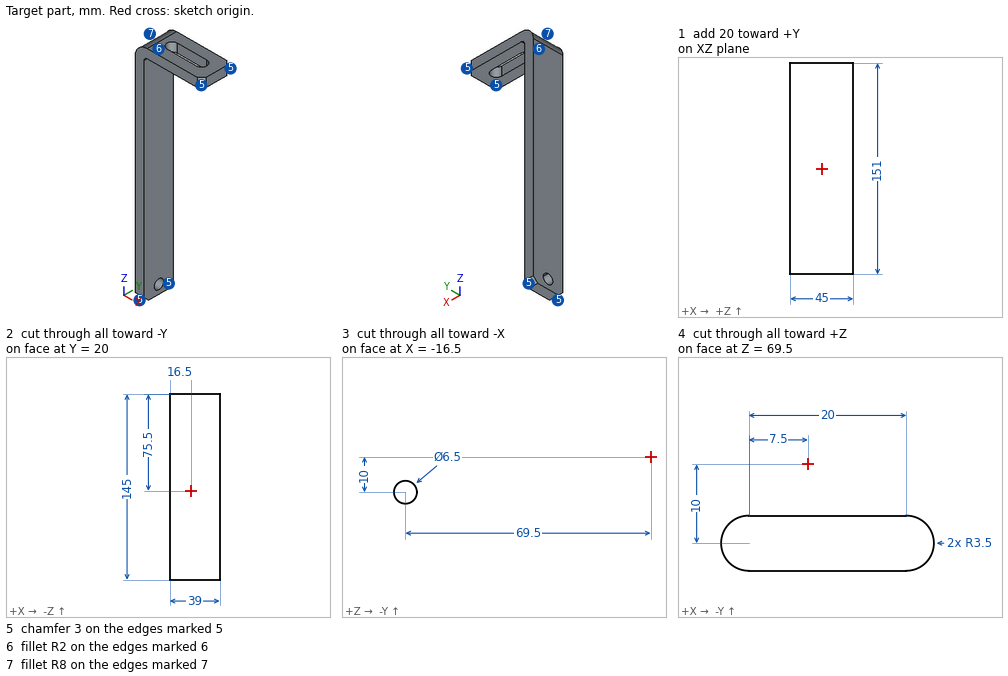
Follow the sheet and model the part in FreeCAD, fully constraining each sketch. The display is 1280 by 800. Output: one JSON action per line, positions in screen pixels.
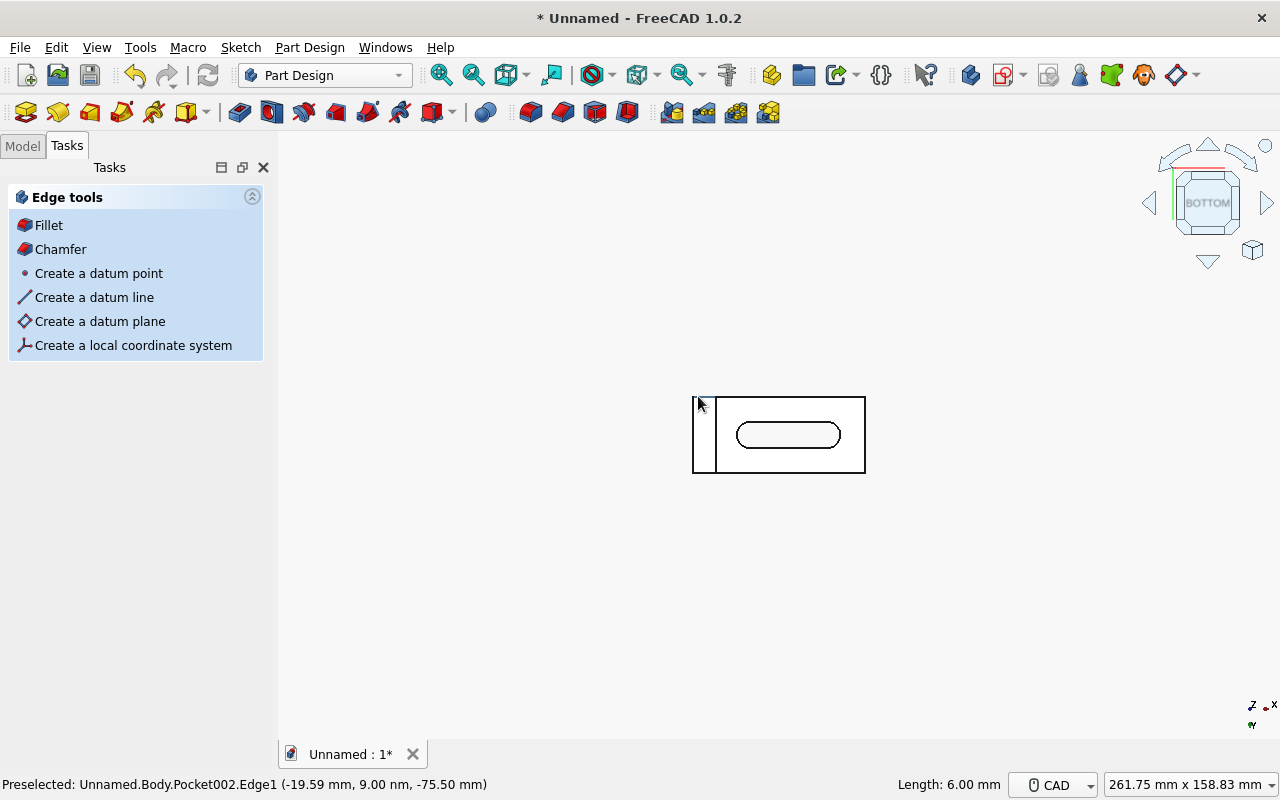
{"action": "key", "text": "0"}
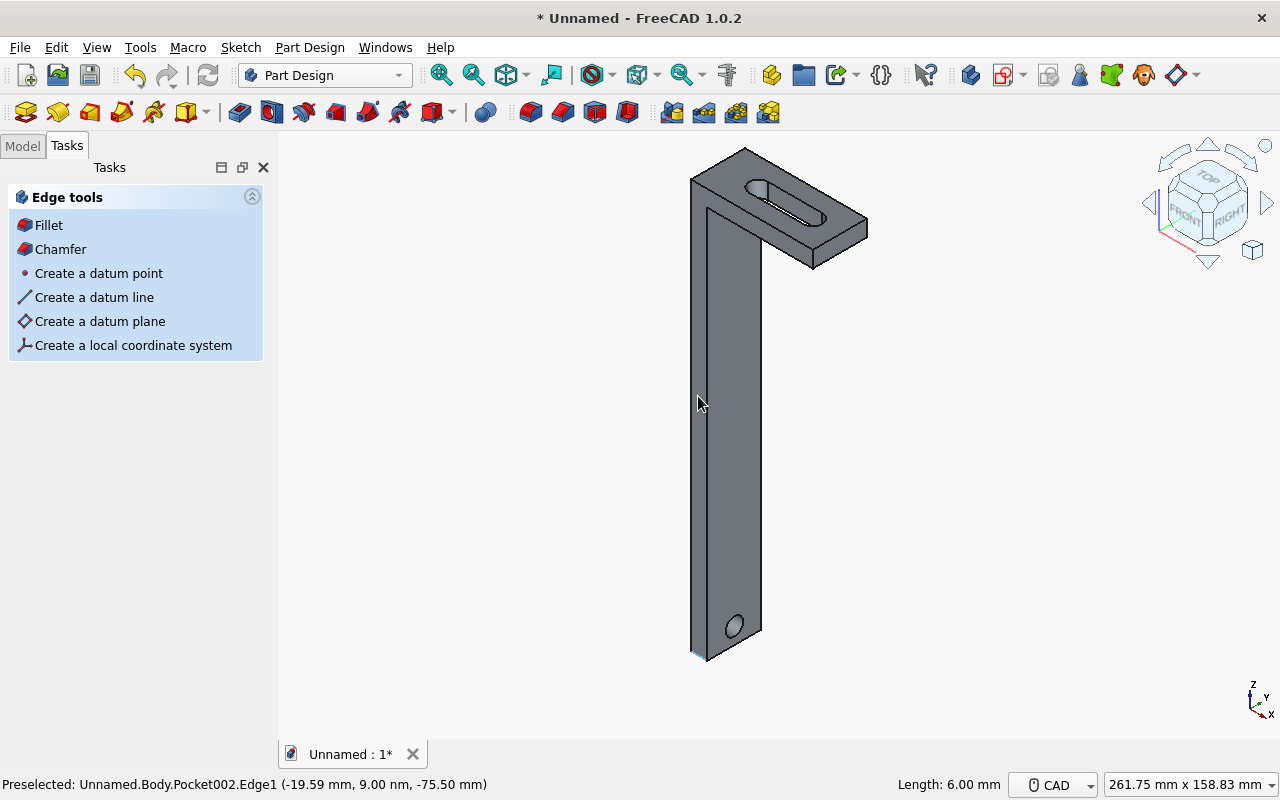
{"action": "left_click", "coordinate": [813, 258], "text": "ctrl"}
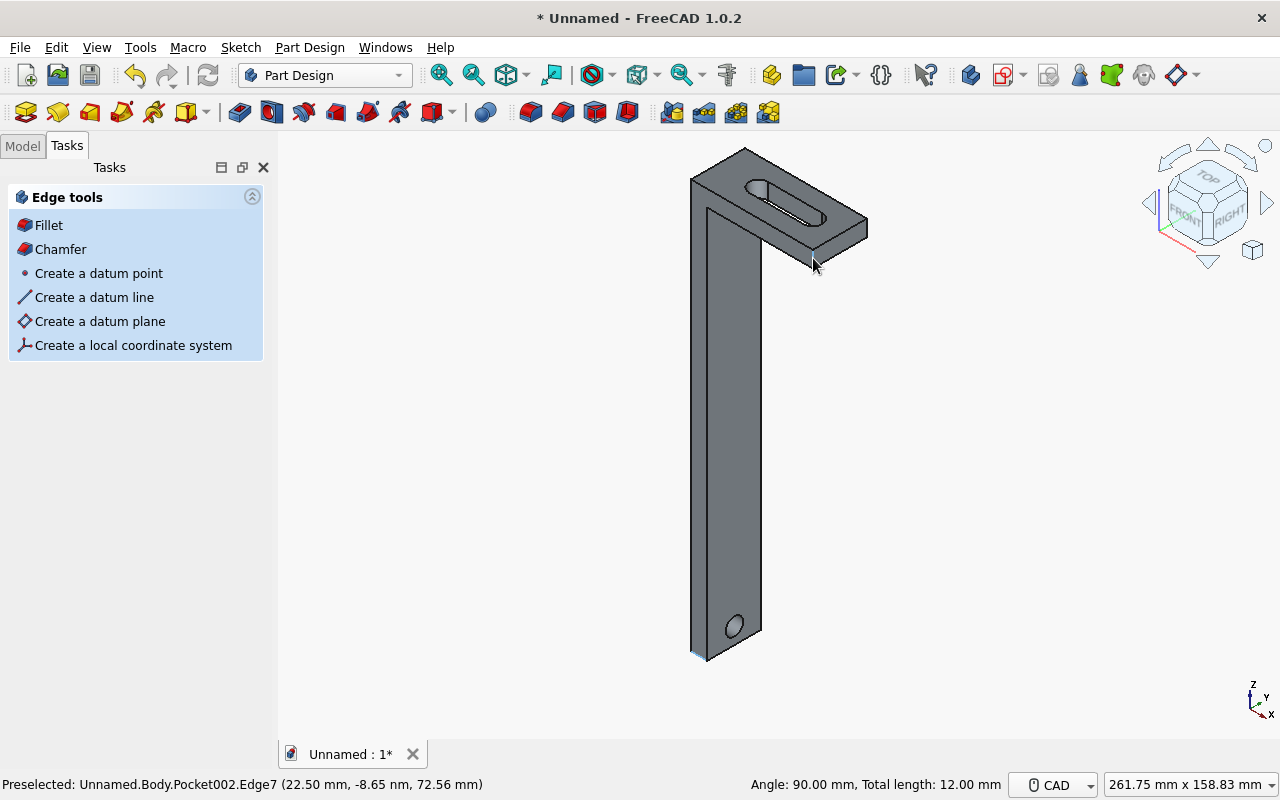
{"action": "key", "text": "2"}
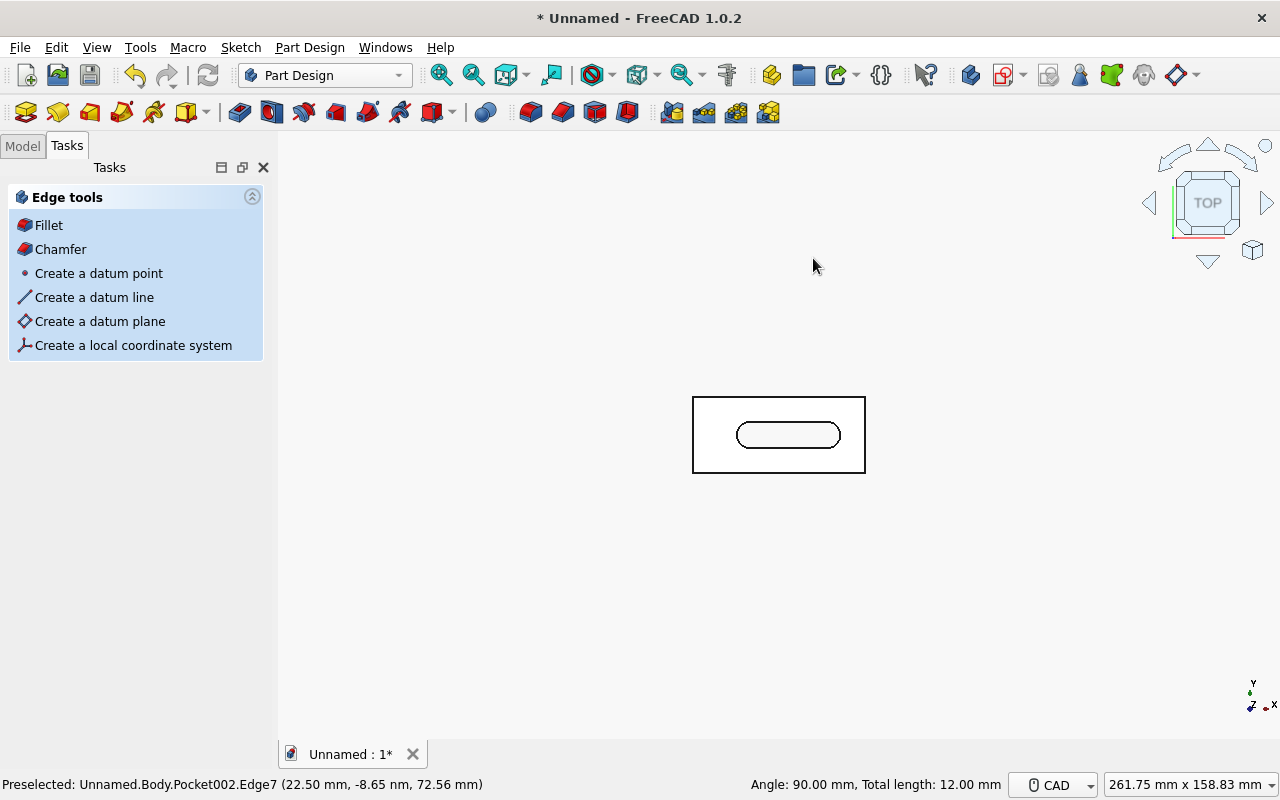
{"action": "left_click", "coordinate": [442, 76]}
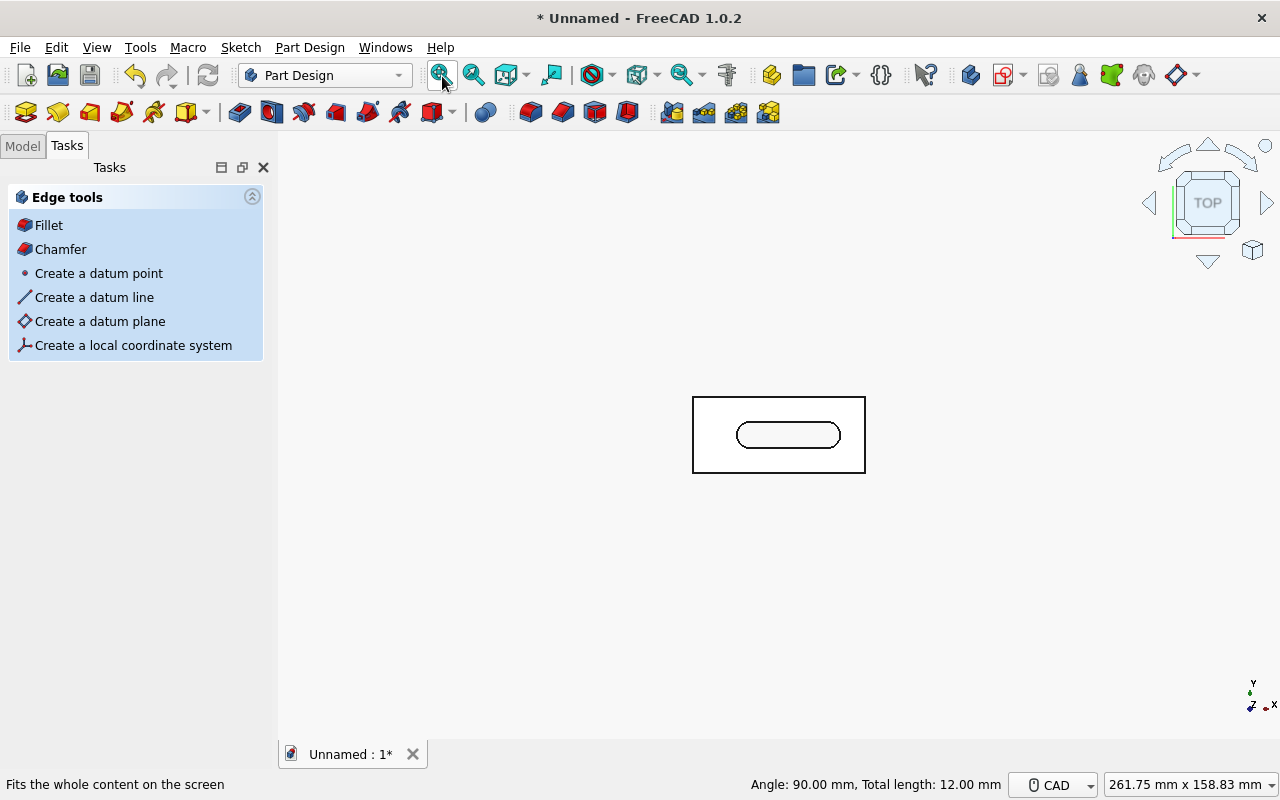
{"action": "key", "text": "1"}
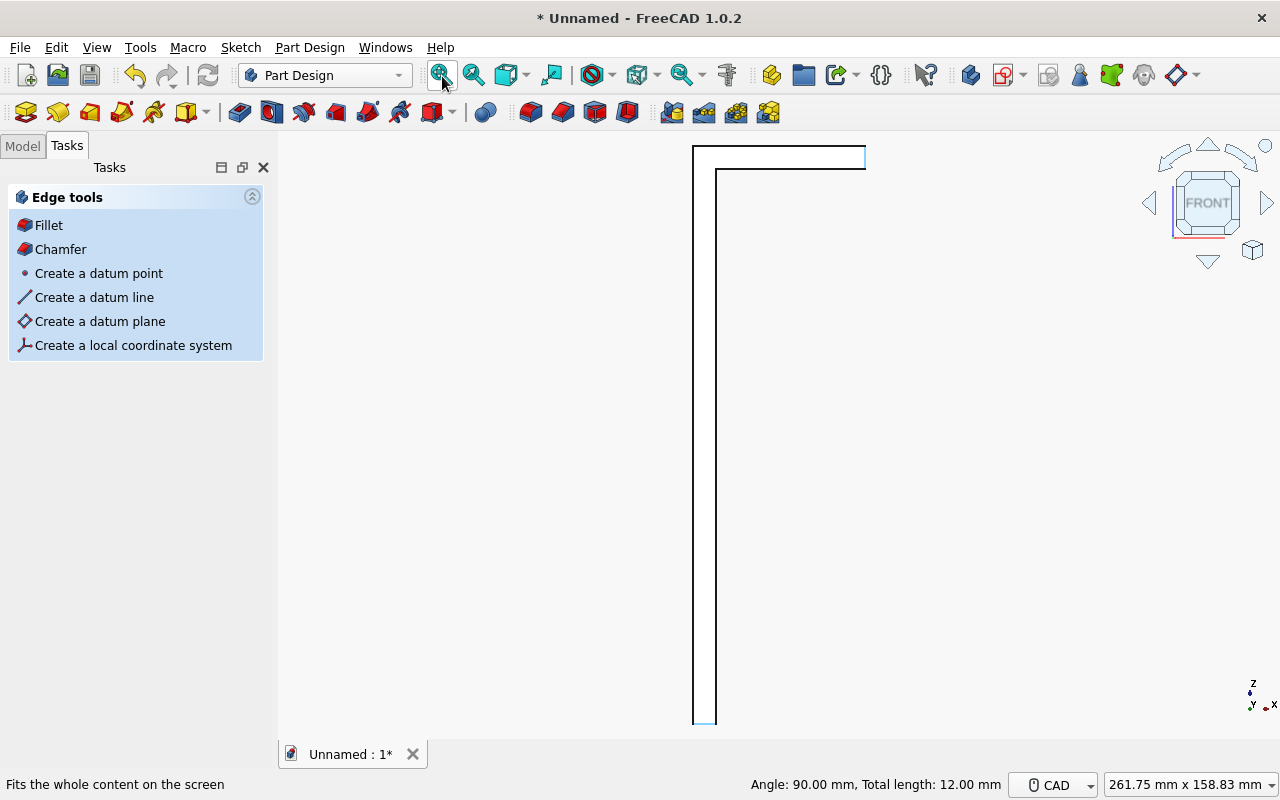
{"action": "key", "text": "3"}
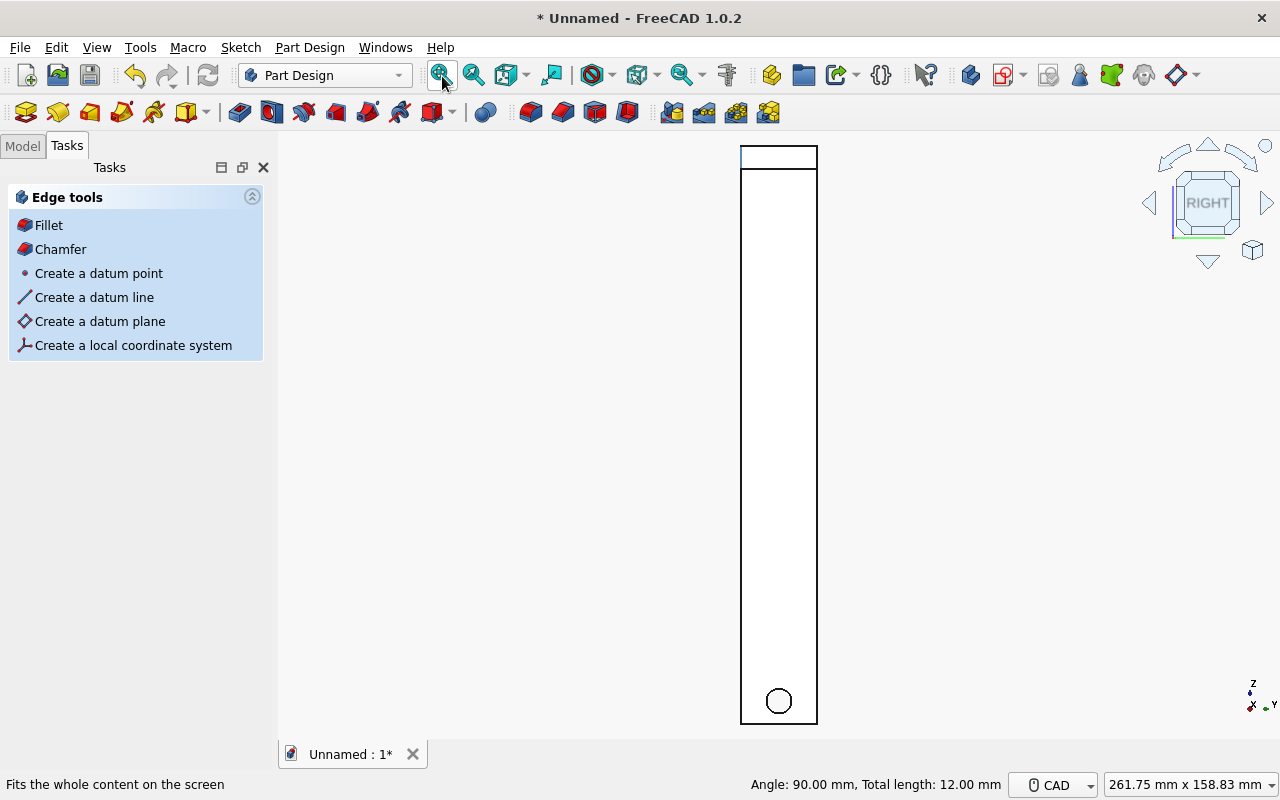
{"action": "left_click", "coordinate": [817, 161], "text": "ctrl"}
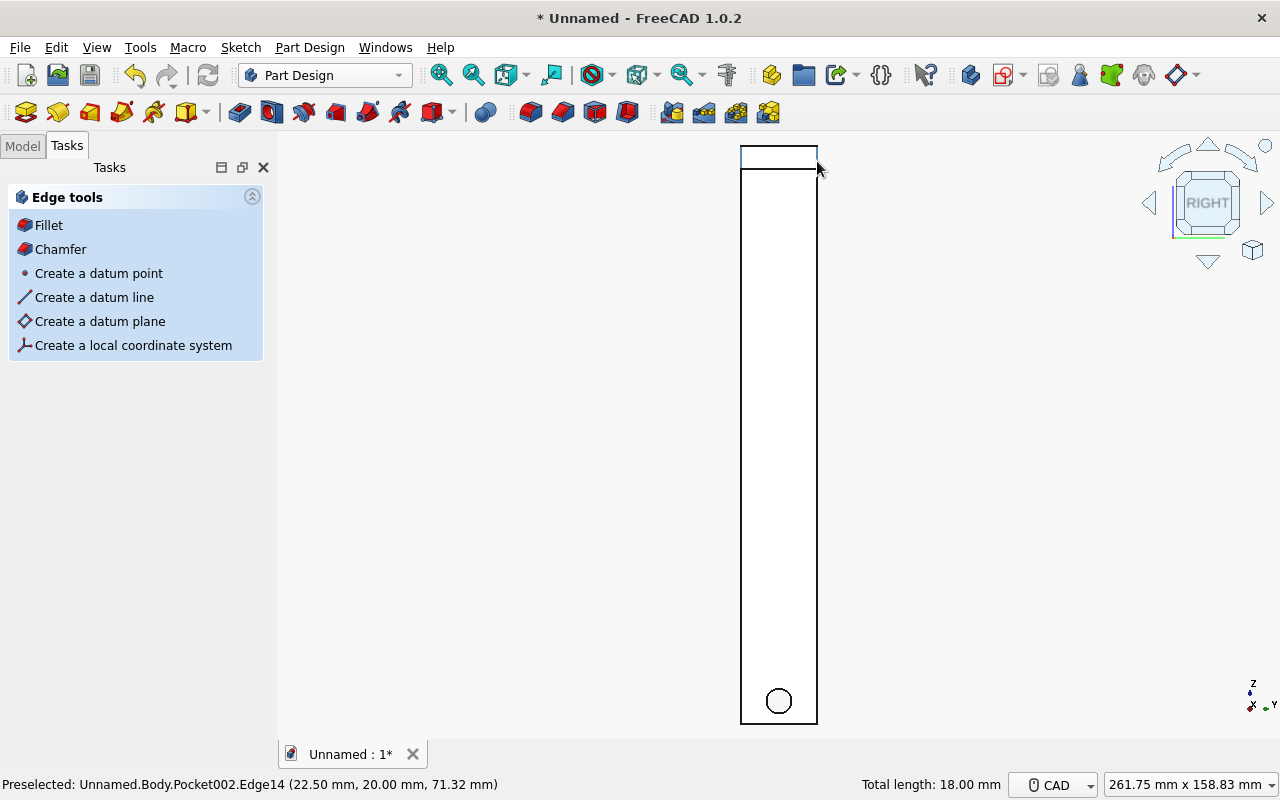
{"action": "key", "text": "5"}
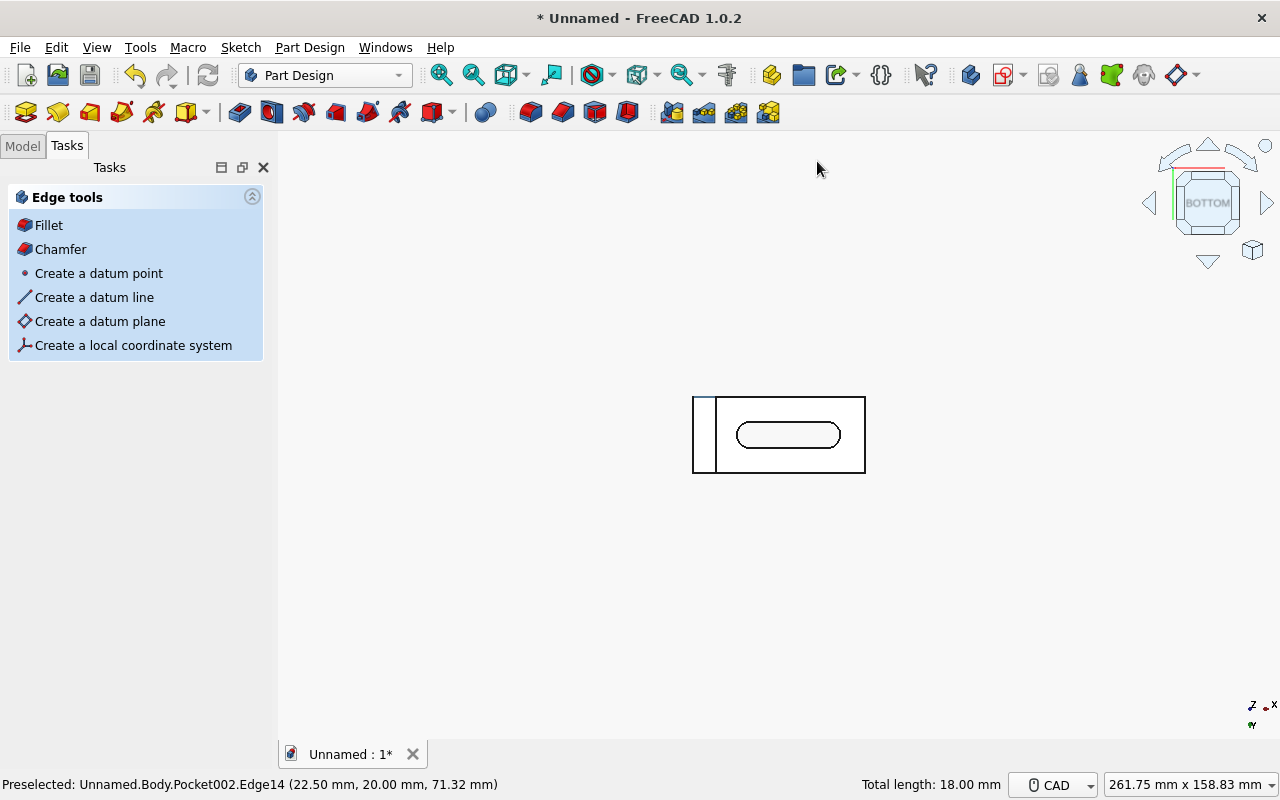
{"action": "left_click", "coordinate": [442, 76]}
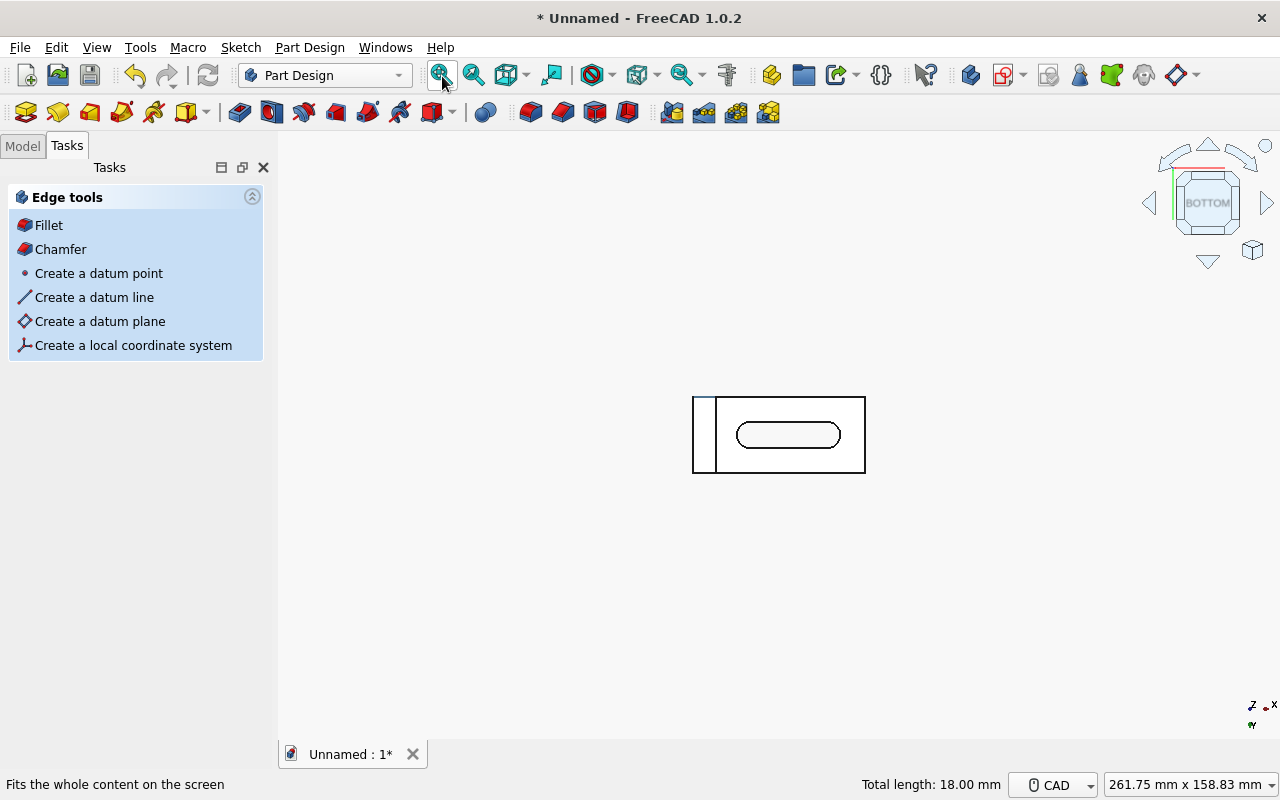
{"action": "key", "text": "4"}